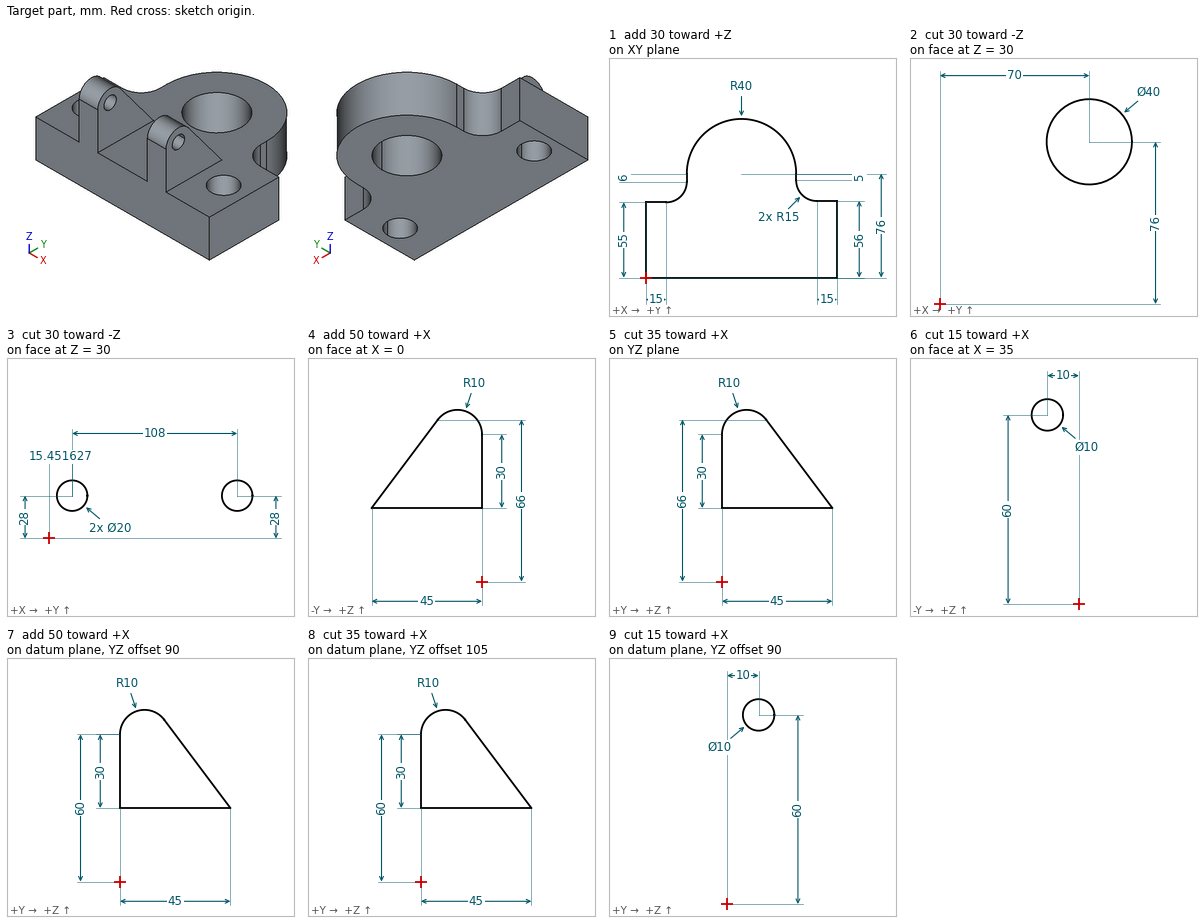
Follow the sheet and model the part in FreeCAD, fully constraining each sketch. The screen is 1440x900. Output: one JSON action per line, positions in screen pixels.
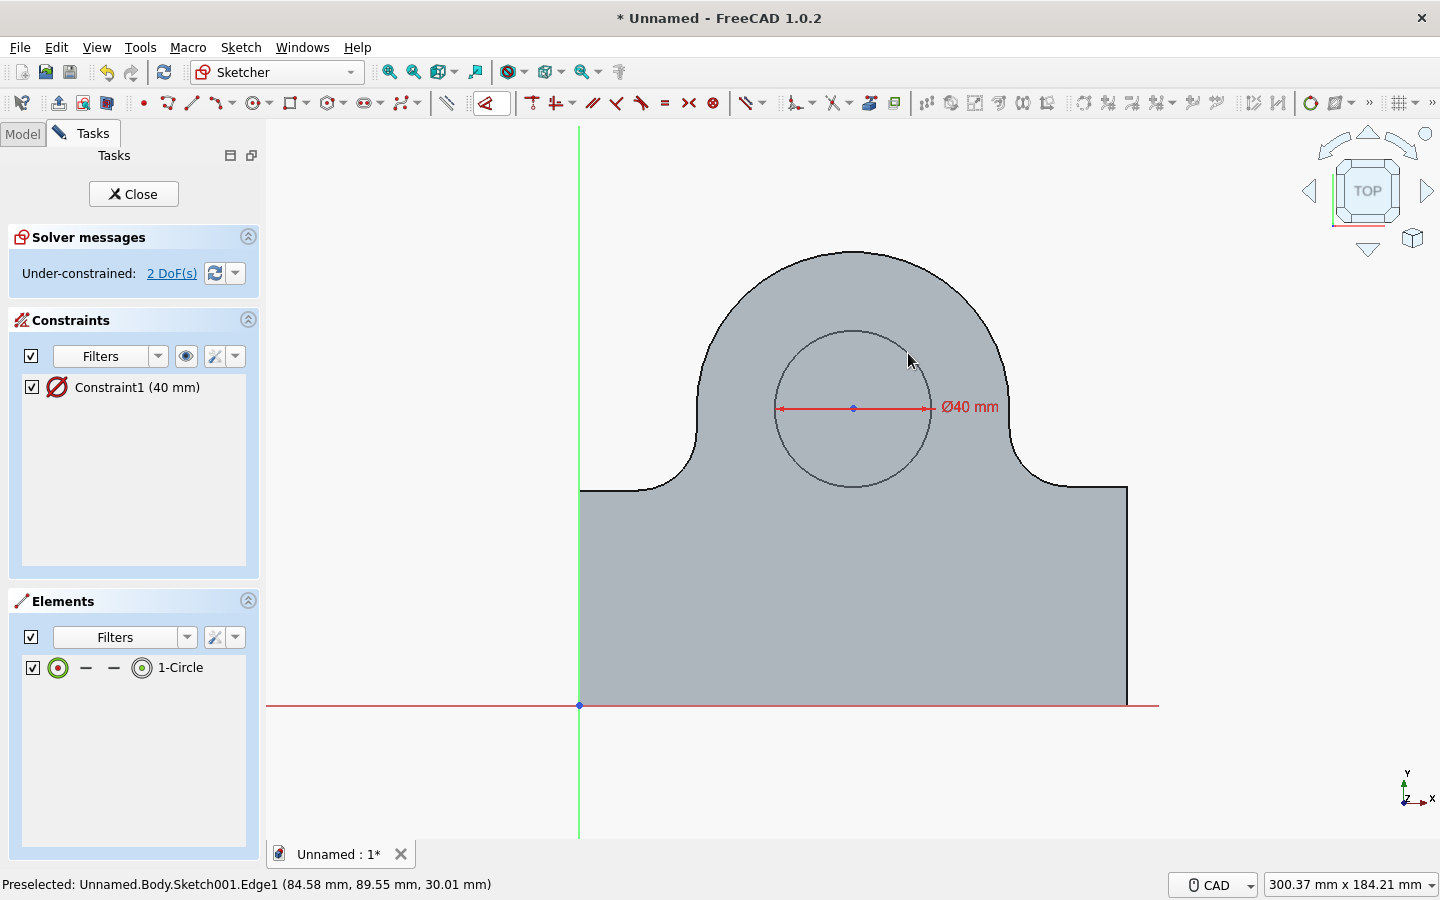
{"action": "left_click", "coordinate": [853, 409]}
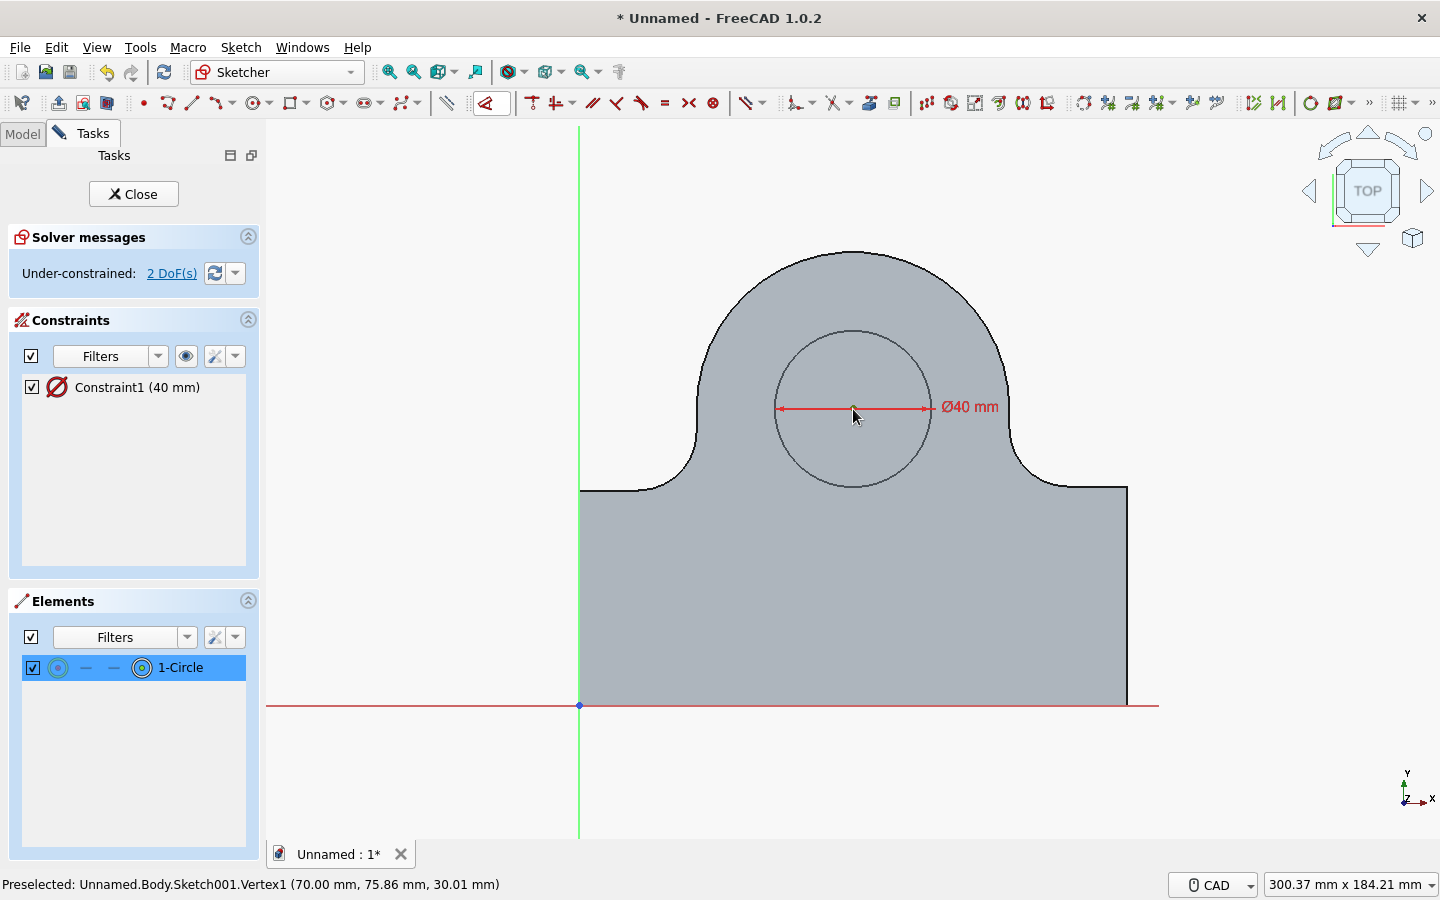
{"action": "key", "text": "l"}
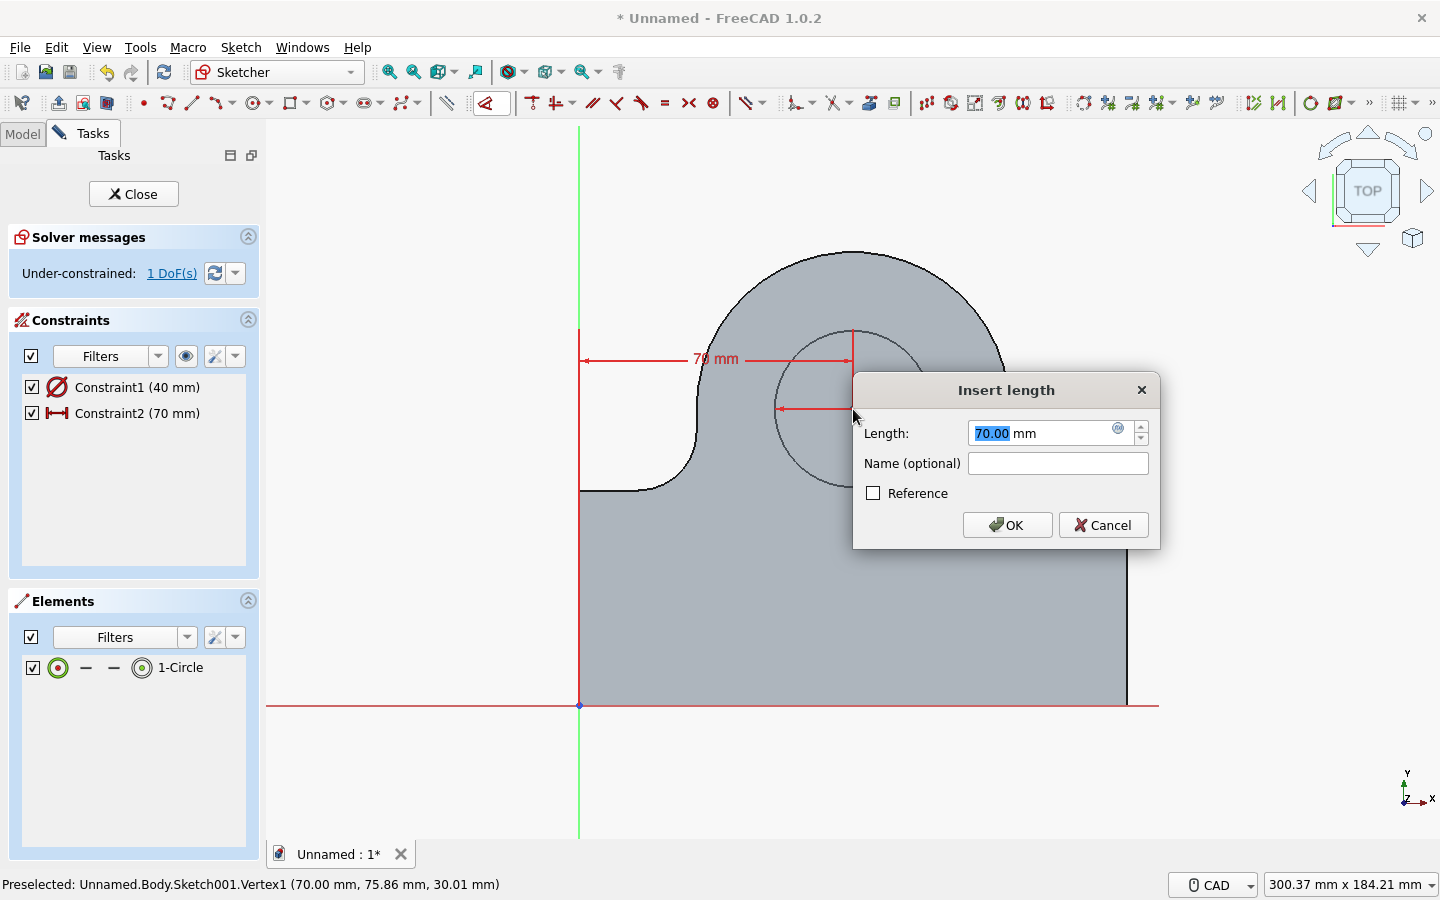
{"action": "type", "text": "70"}
{"action": "key", "text": "Return"}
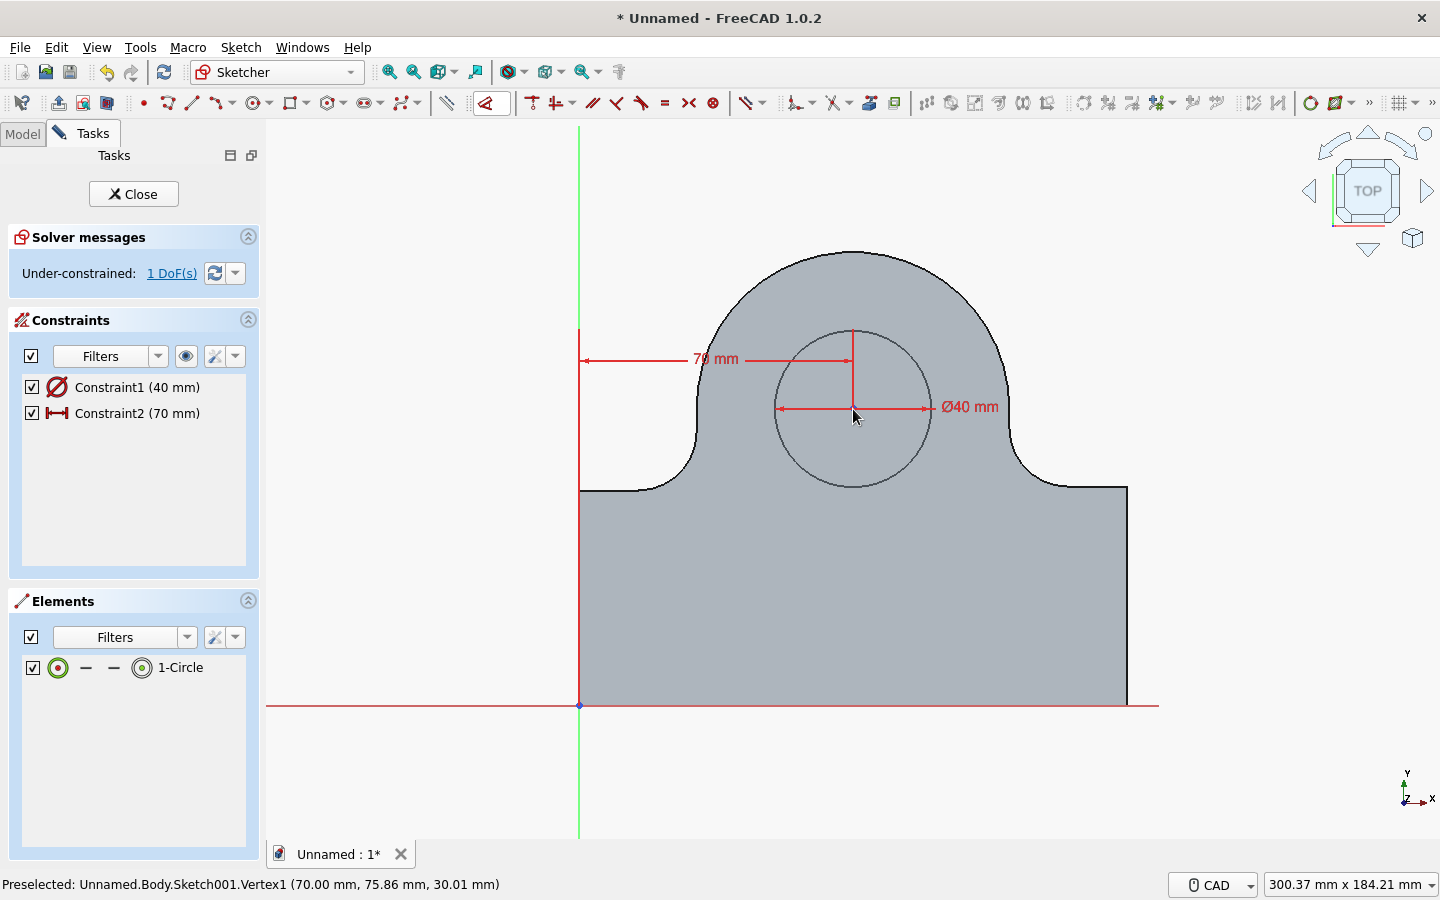
{"action": "left_click", "coordinate": [853, 409]}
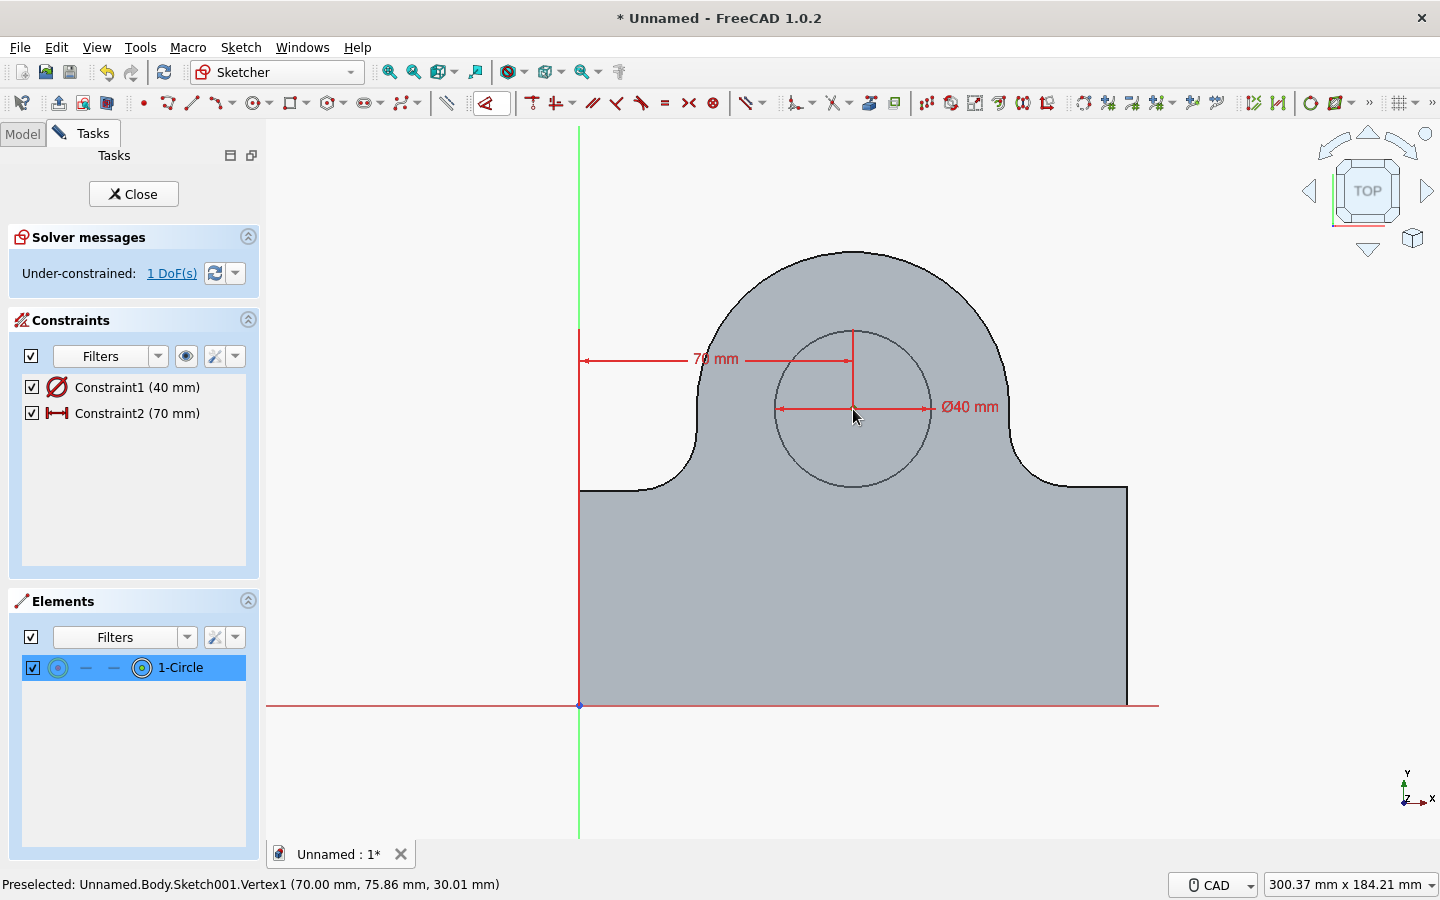
{"action": "key", "text": "i"}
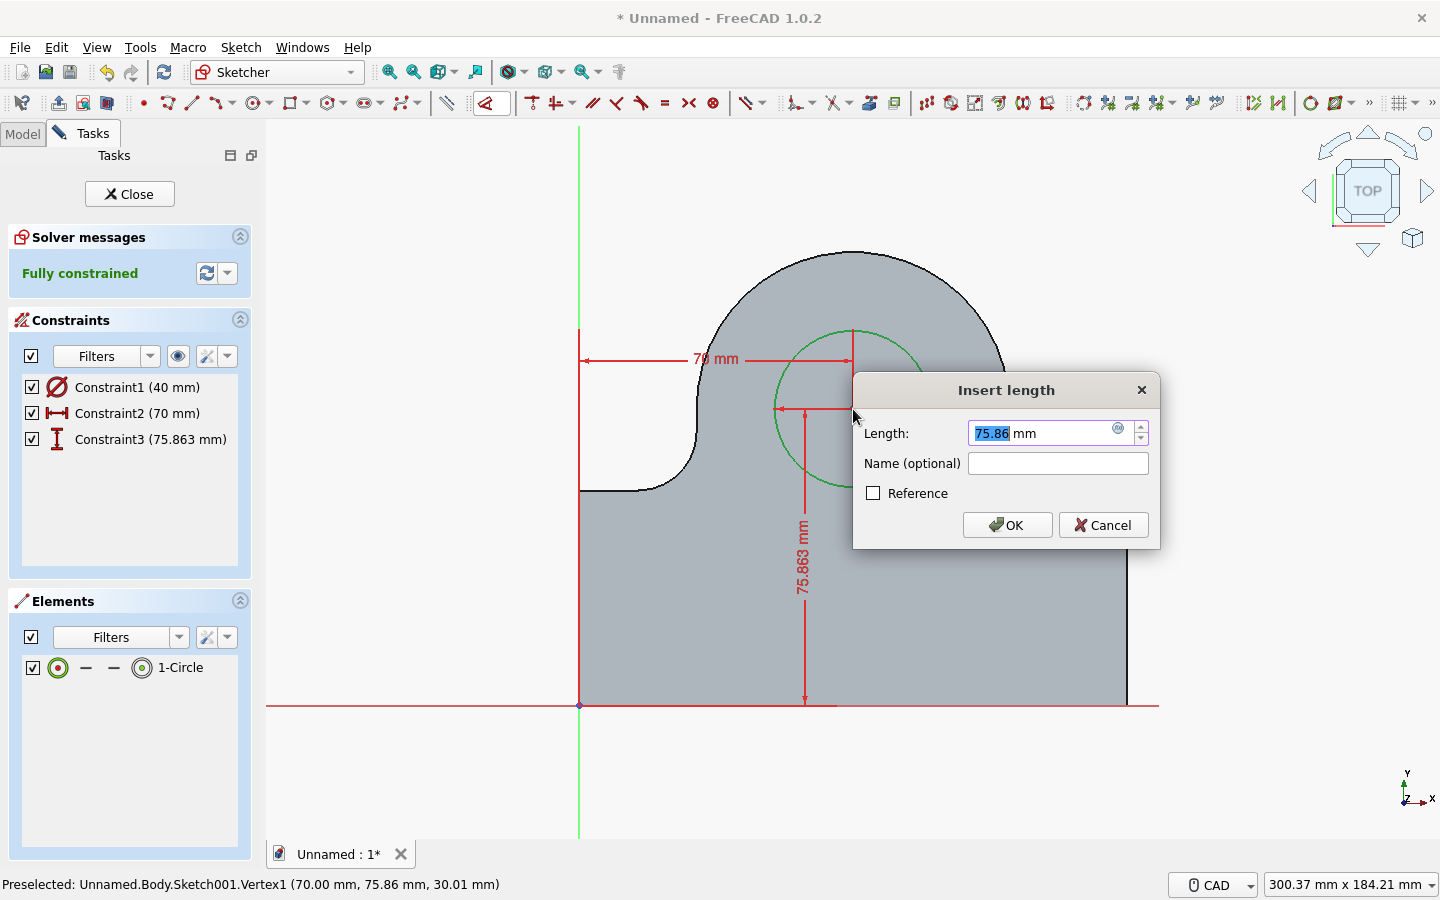
{"action": "type", "text": "76"}
{"action": "key", "text": "Return"}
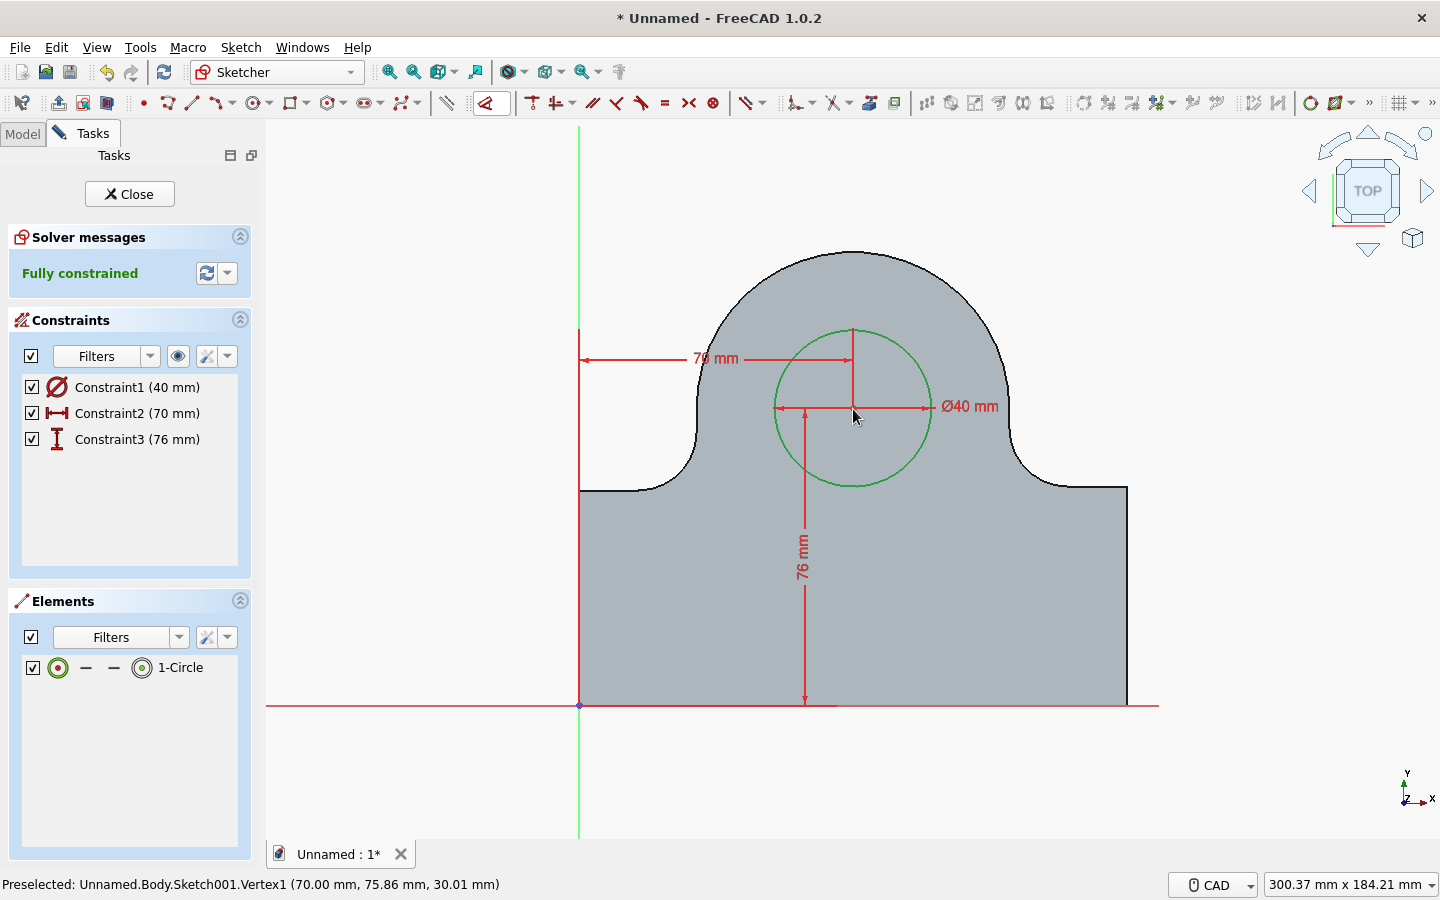
{"action": "left_click", "coordinate": [130, 194]}